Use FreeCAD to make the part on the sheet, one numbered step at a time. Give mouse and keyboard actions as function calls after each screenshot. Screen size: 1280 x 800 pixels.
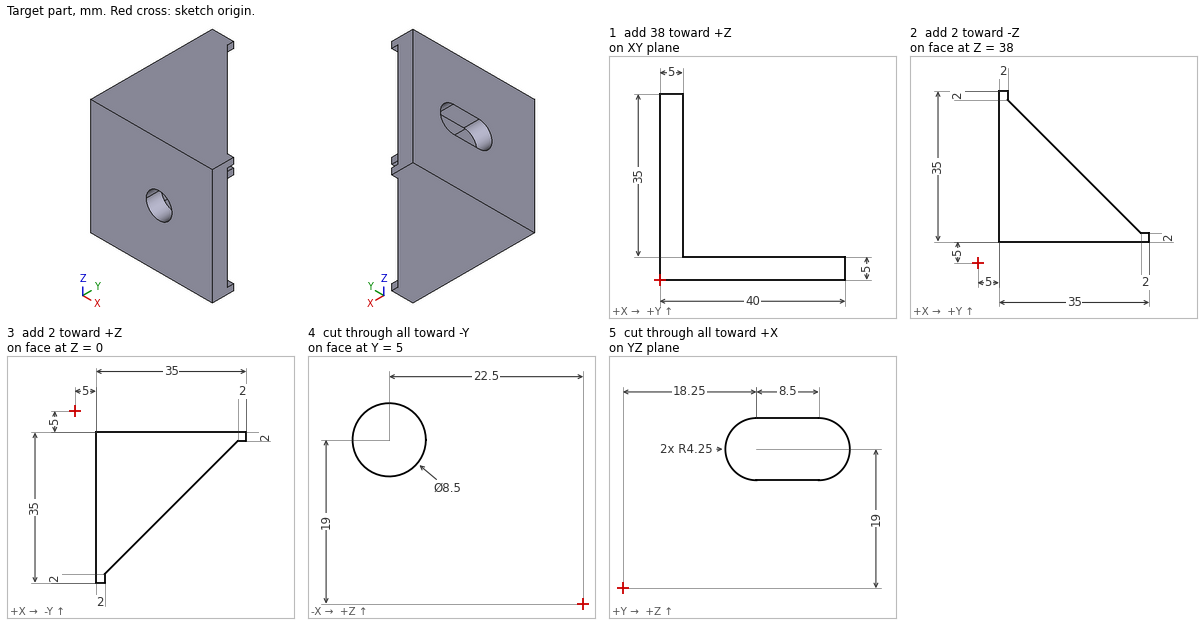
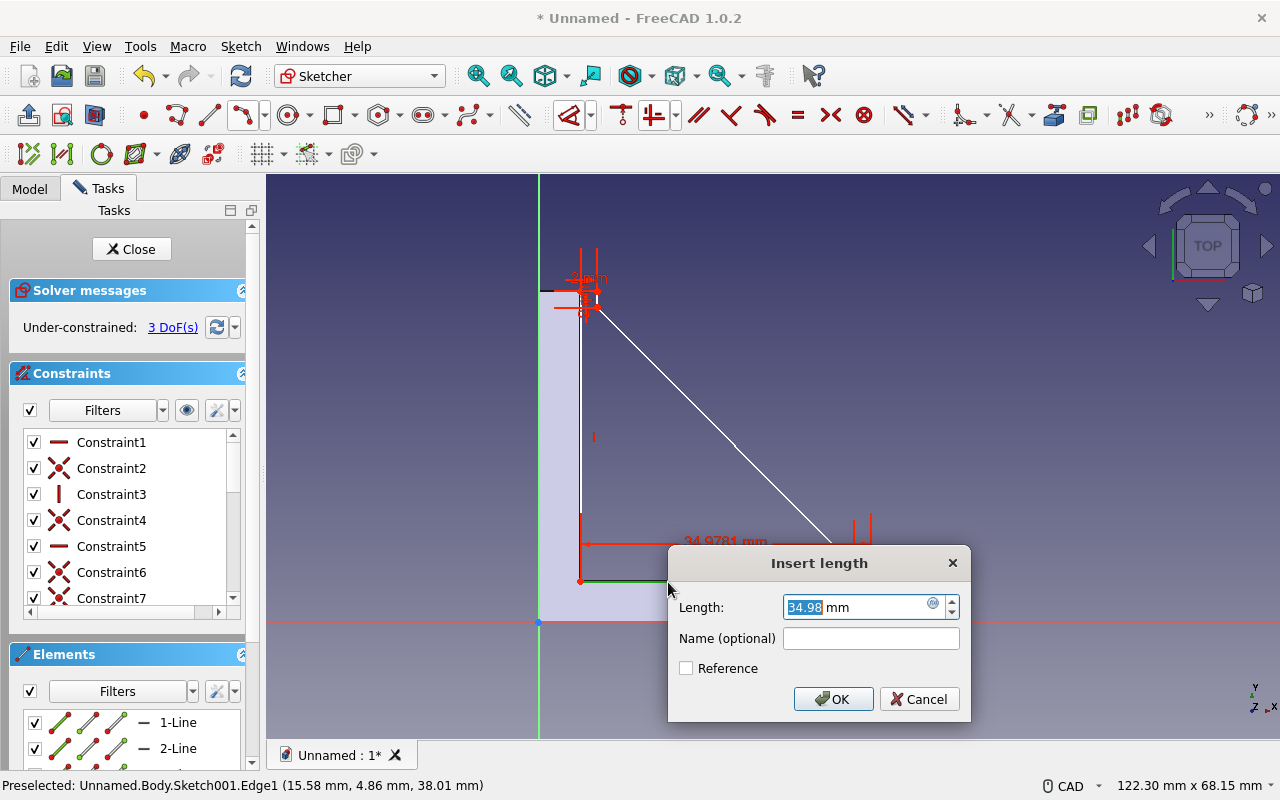
text(35)
key(Return)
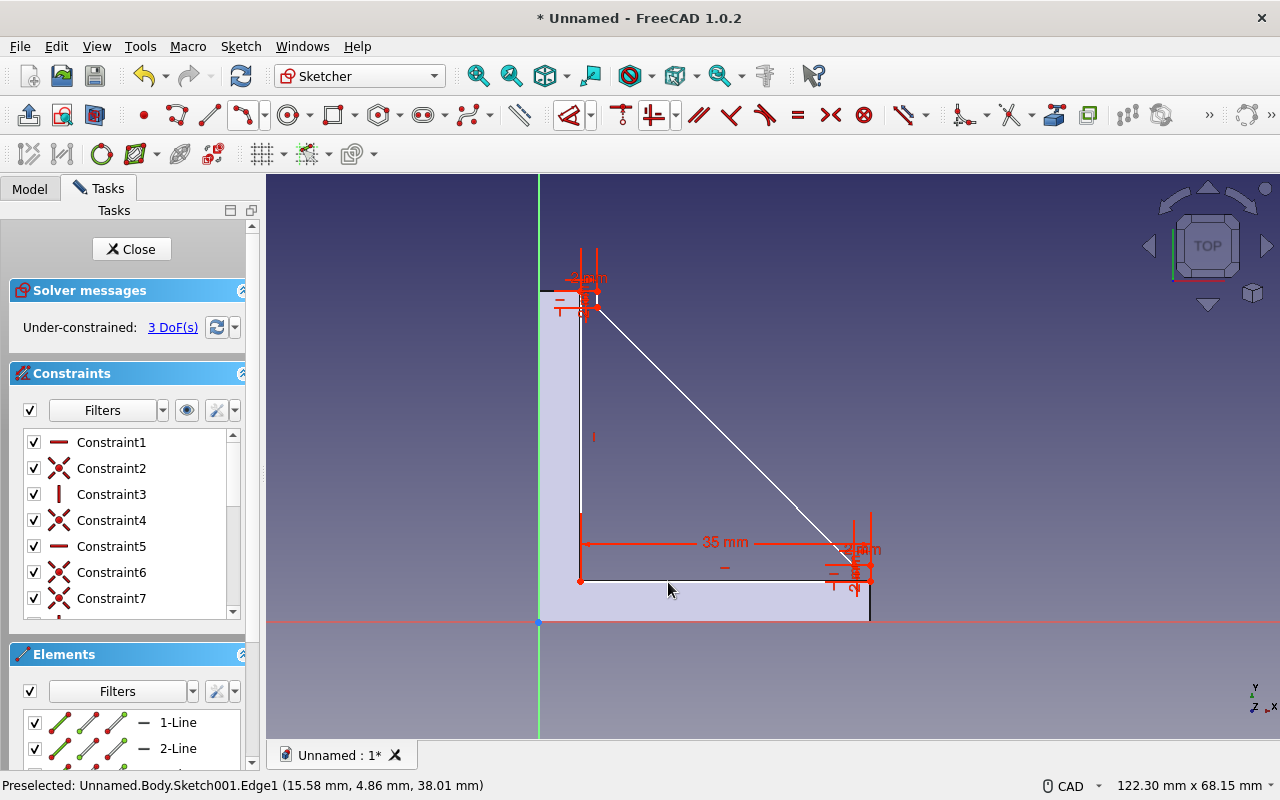
click(581, 379)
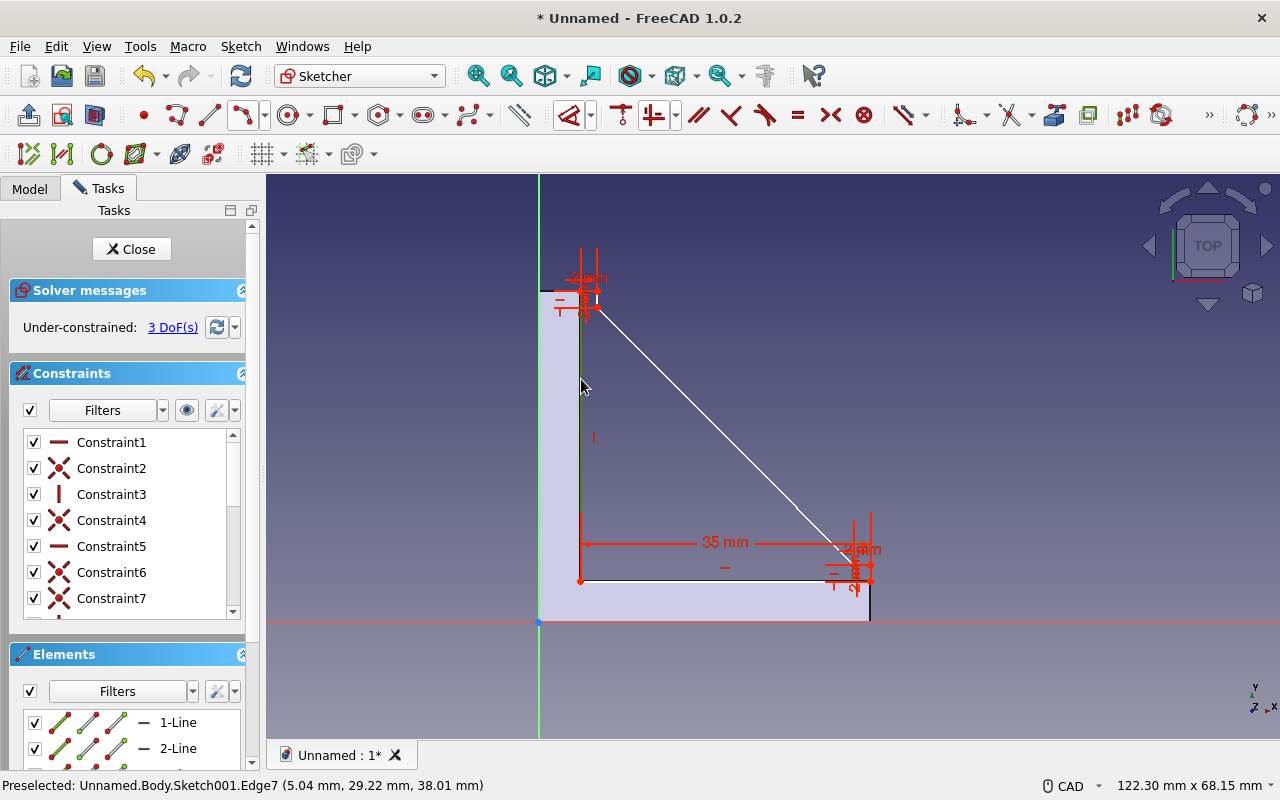
key(i)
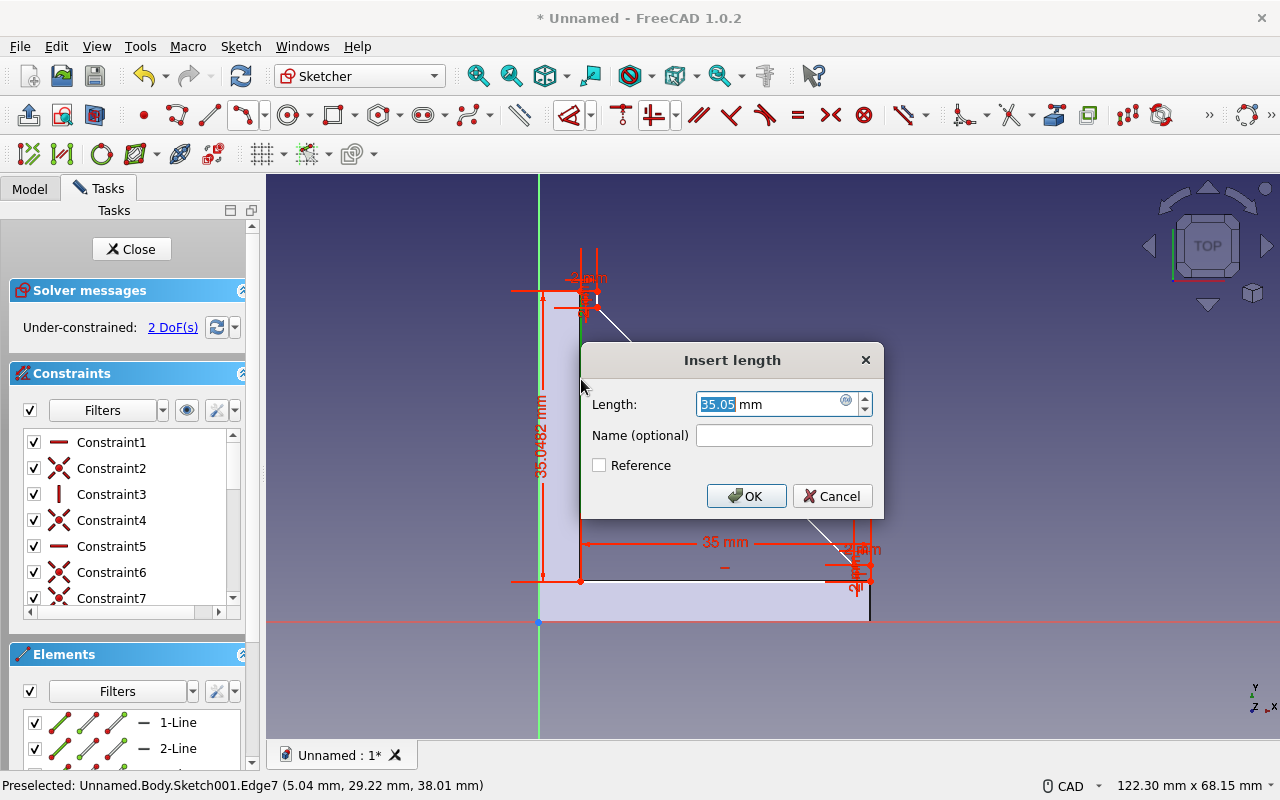
text(35)
key(Return)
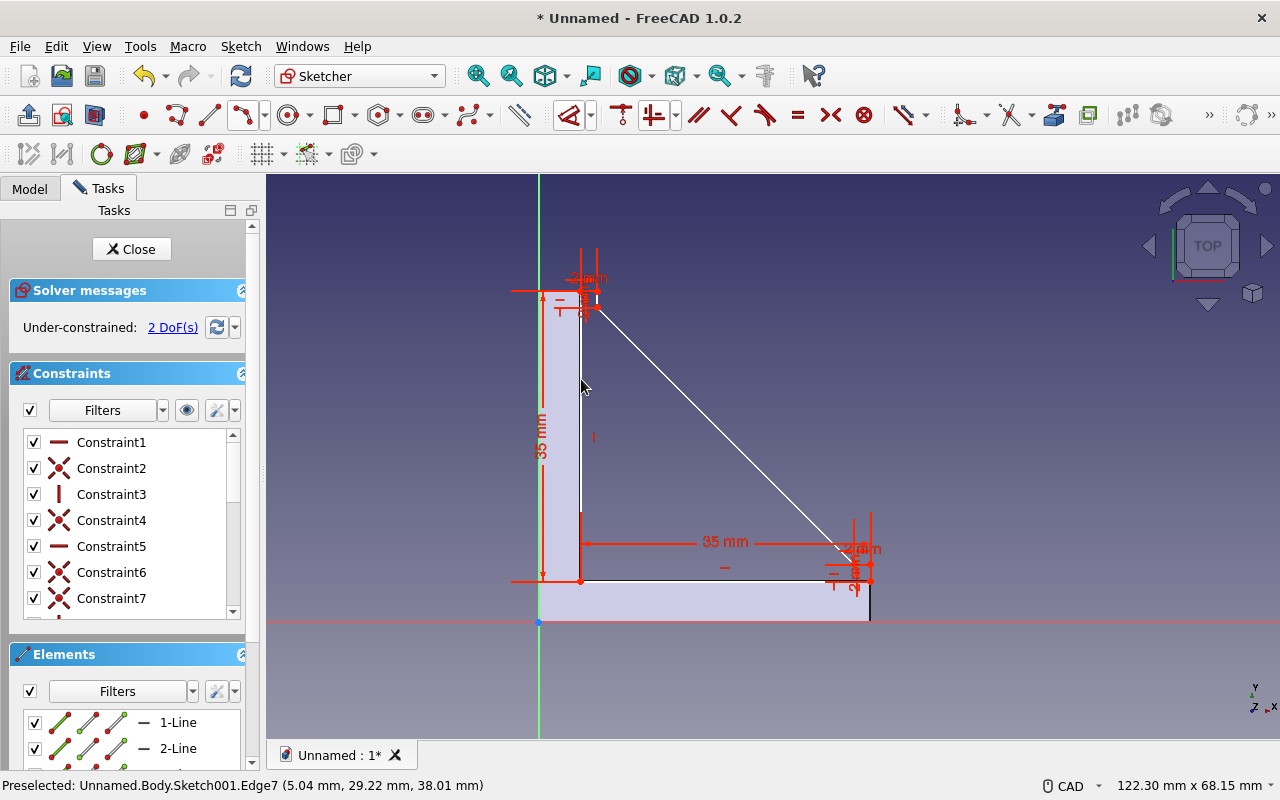
click(581, 582)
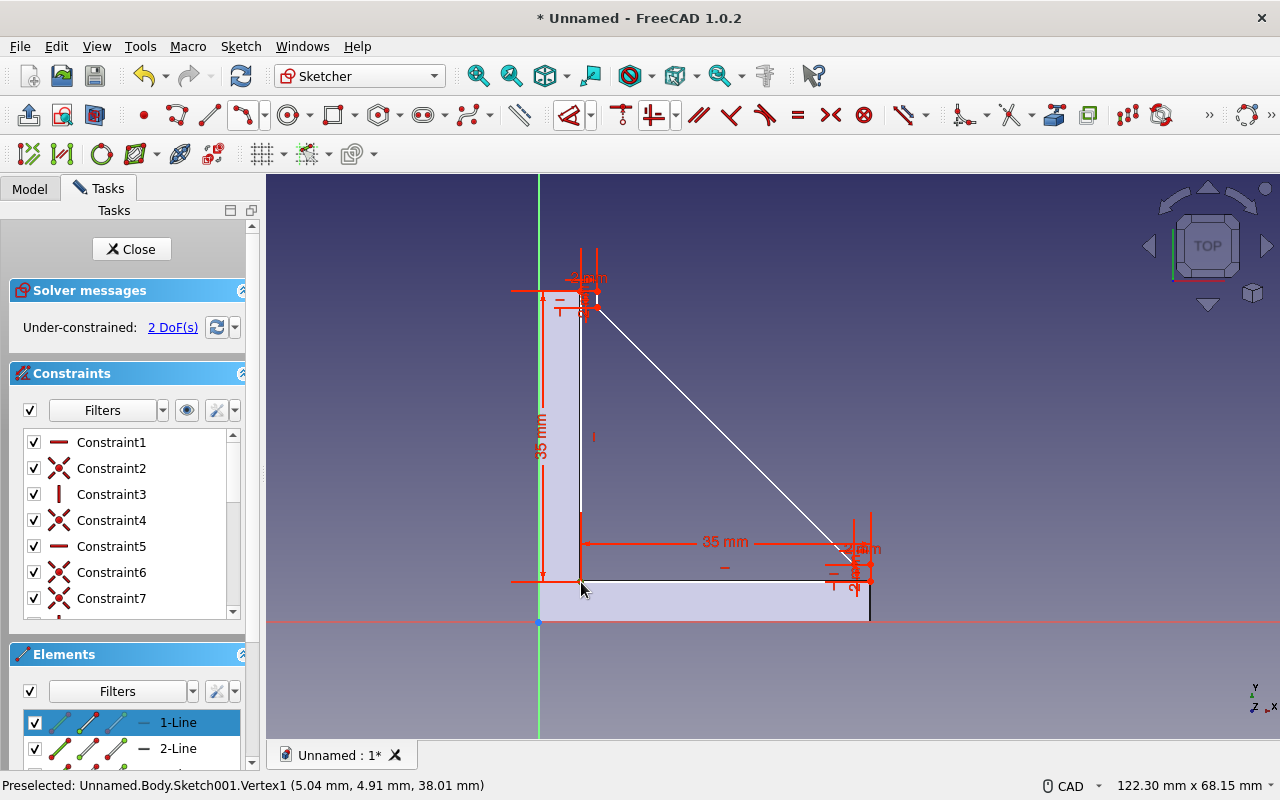
key(l)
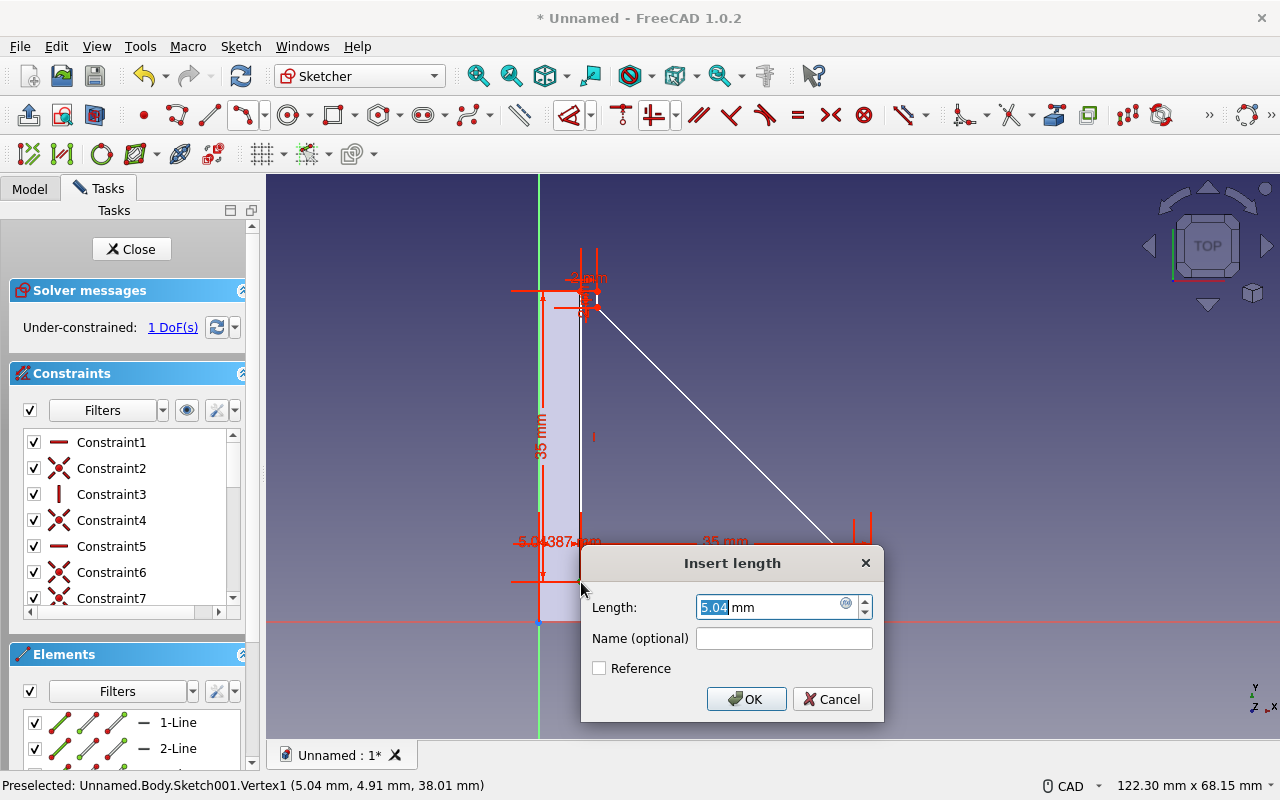
text(5)
key(Return)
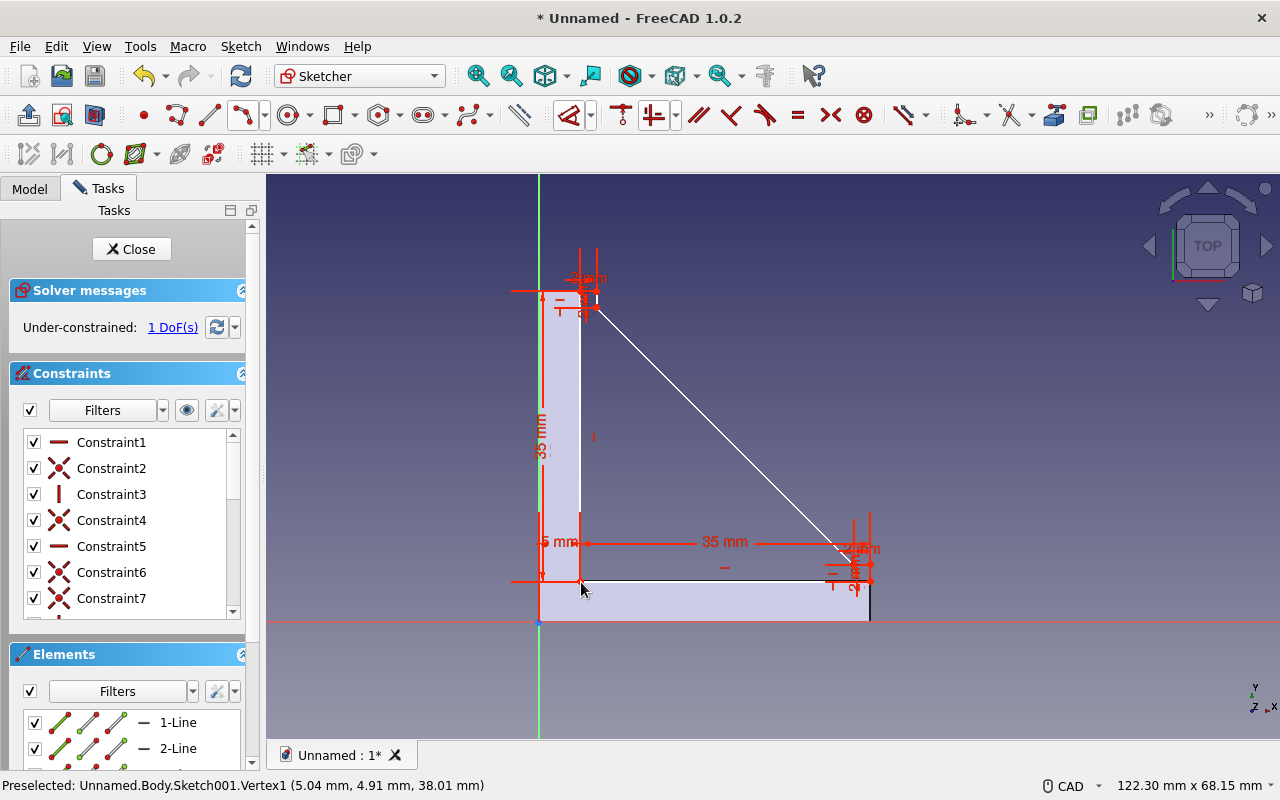
click(580, 582)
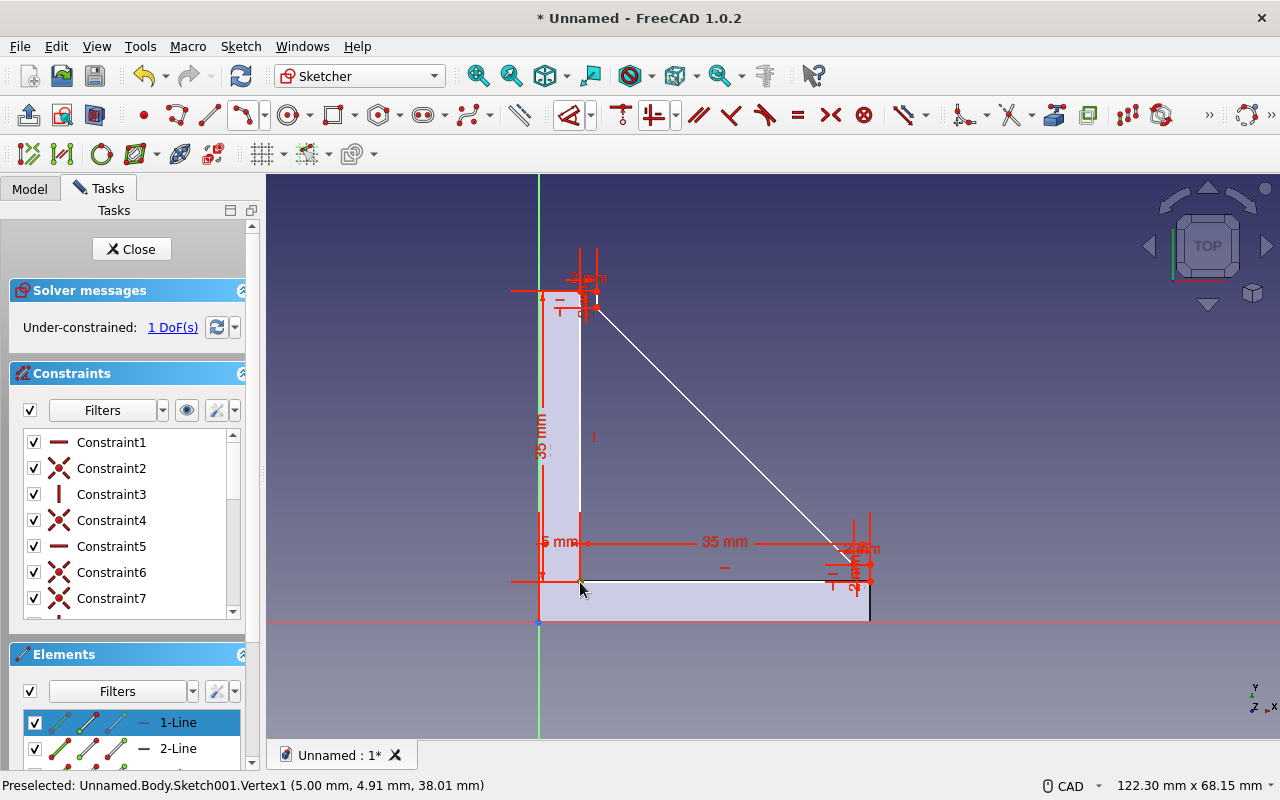
key(i)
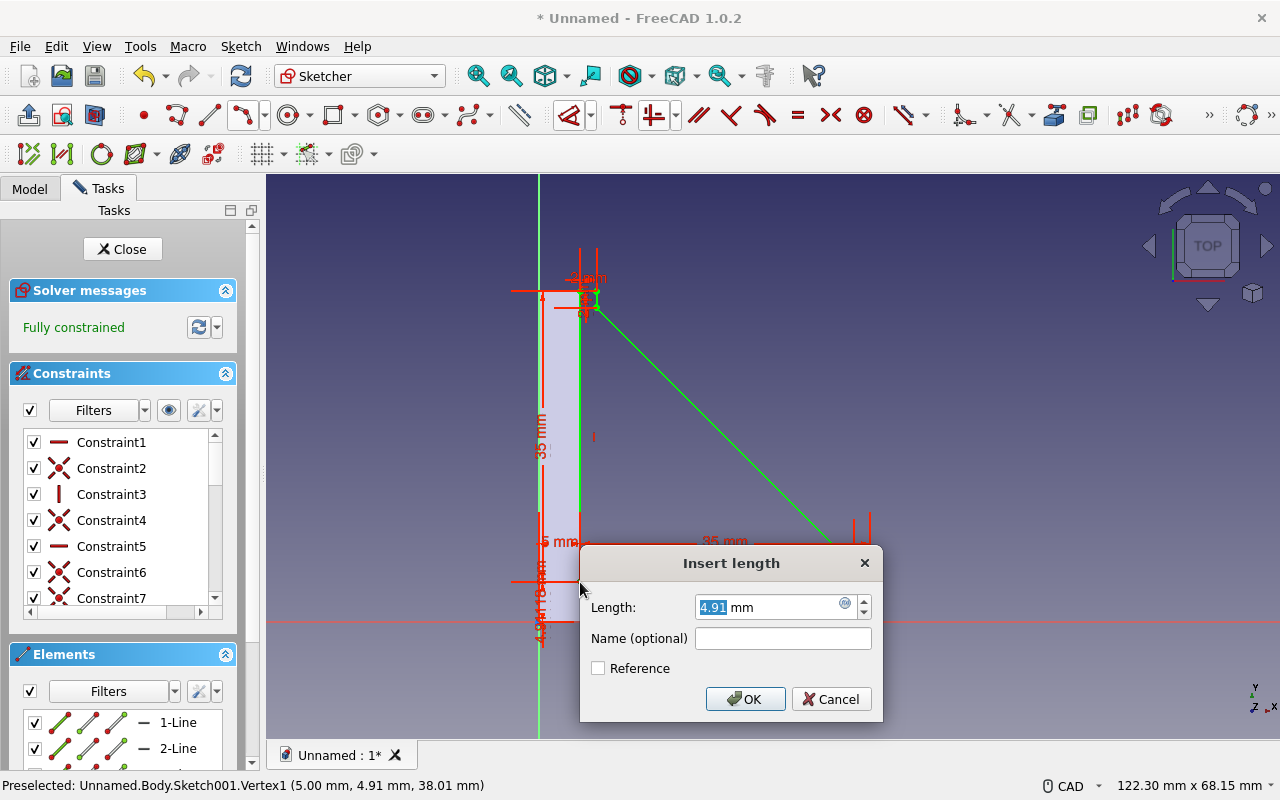
text(5)
key(Return)